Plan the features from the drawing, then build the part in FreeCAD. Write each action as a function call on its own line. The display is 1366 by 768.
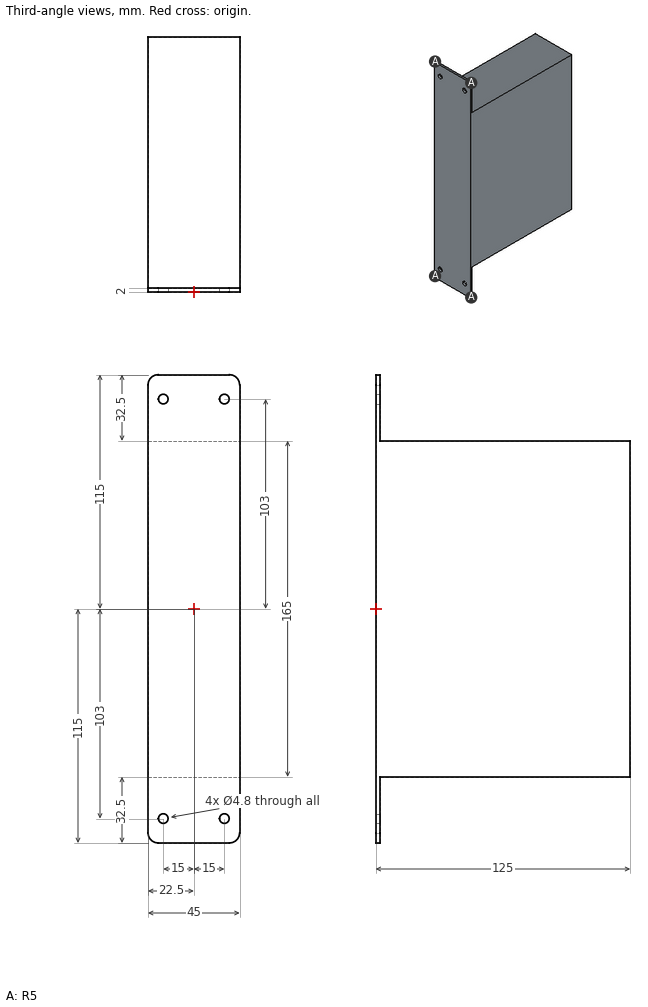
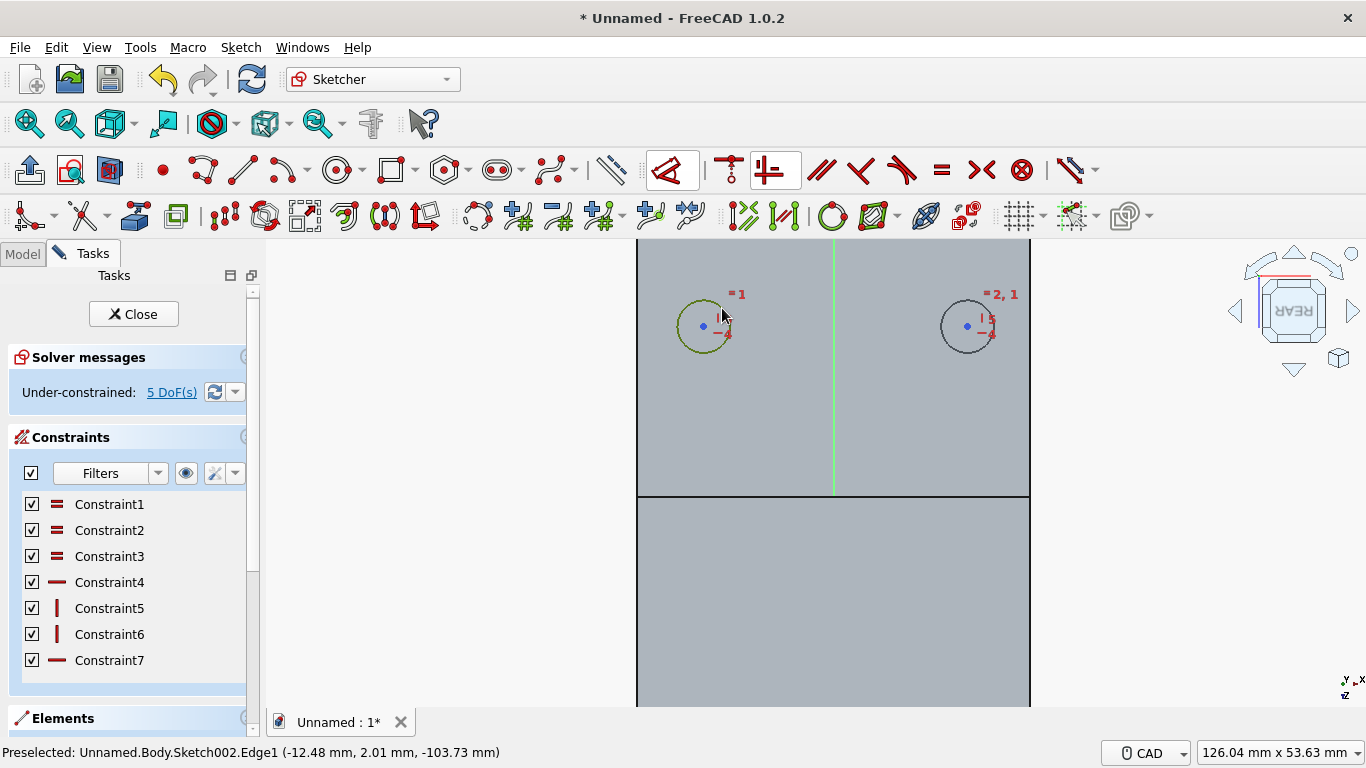
click(694, 170)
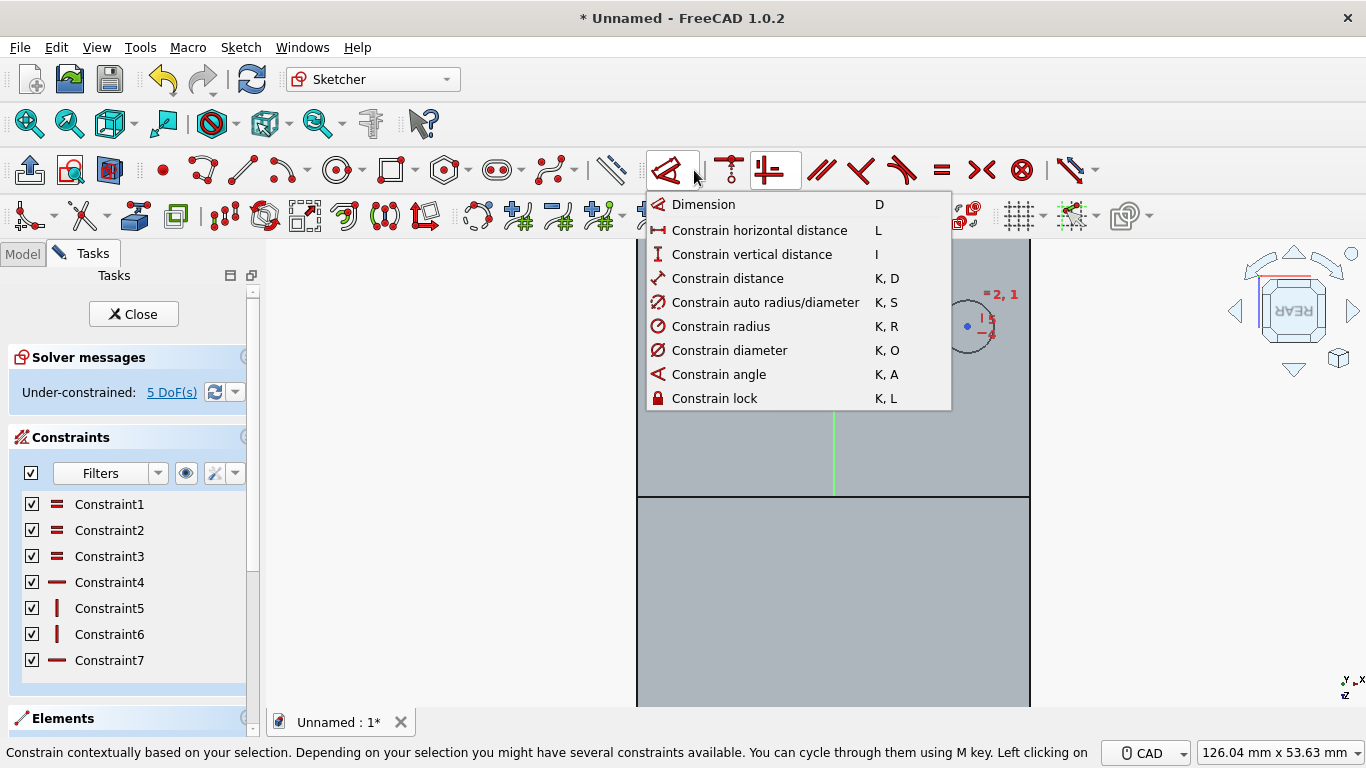
click(799, 350)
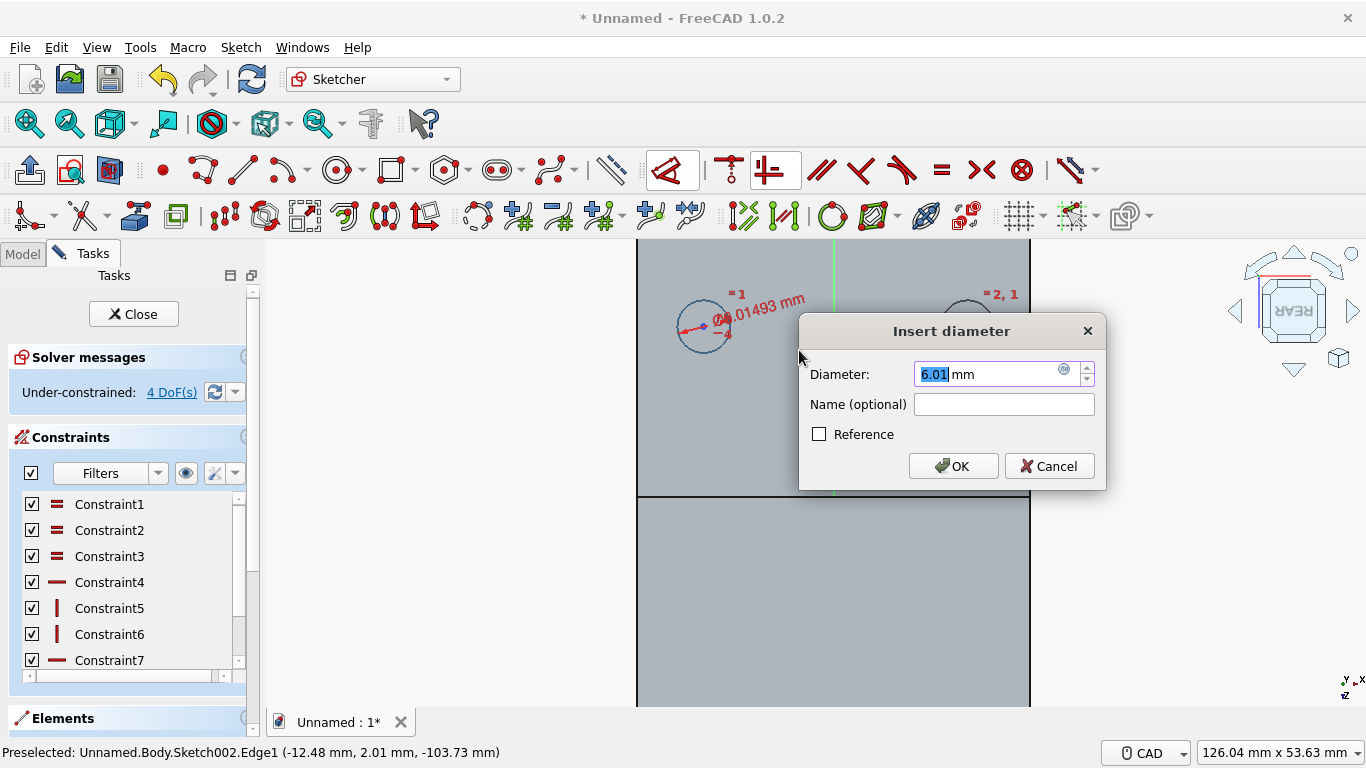
text(4.8)
key(Return)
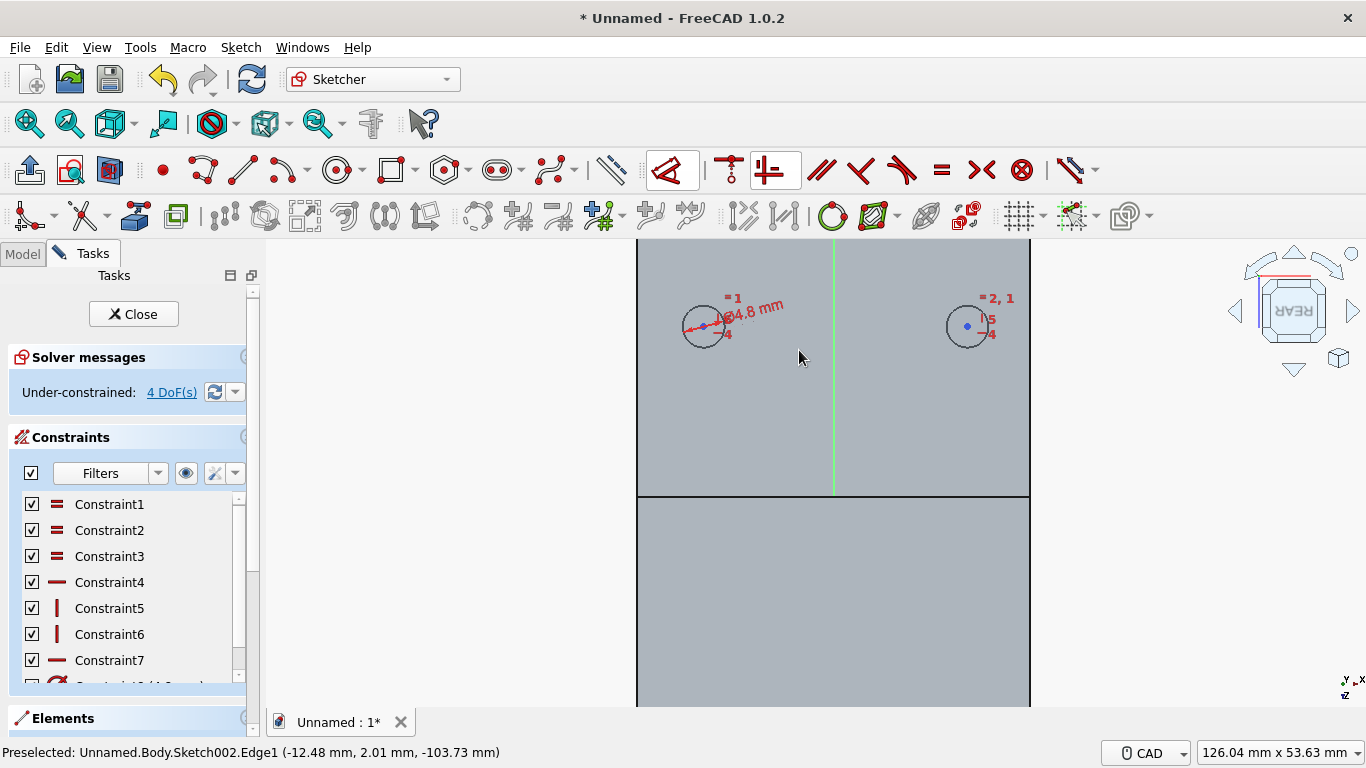
scroll(730, 326, down, 9)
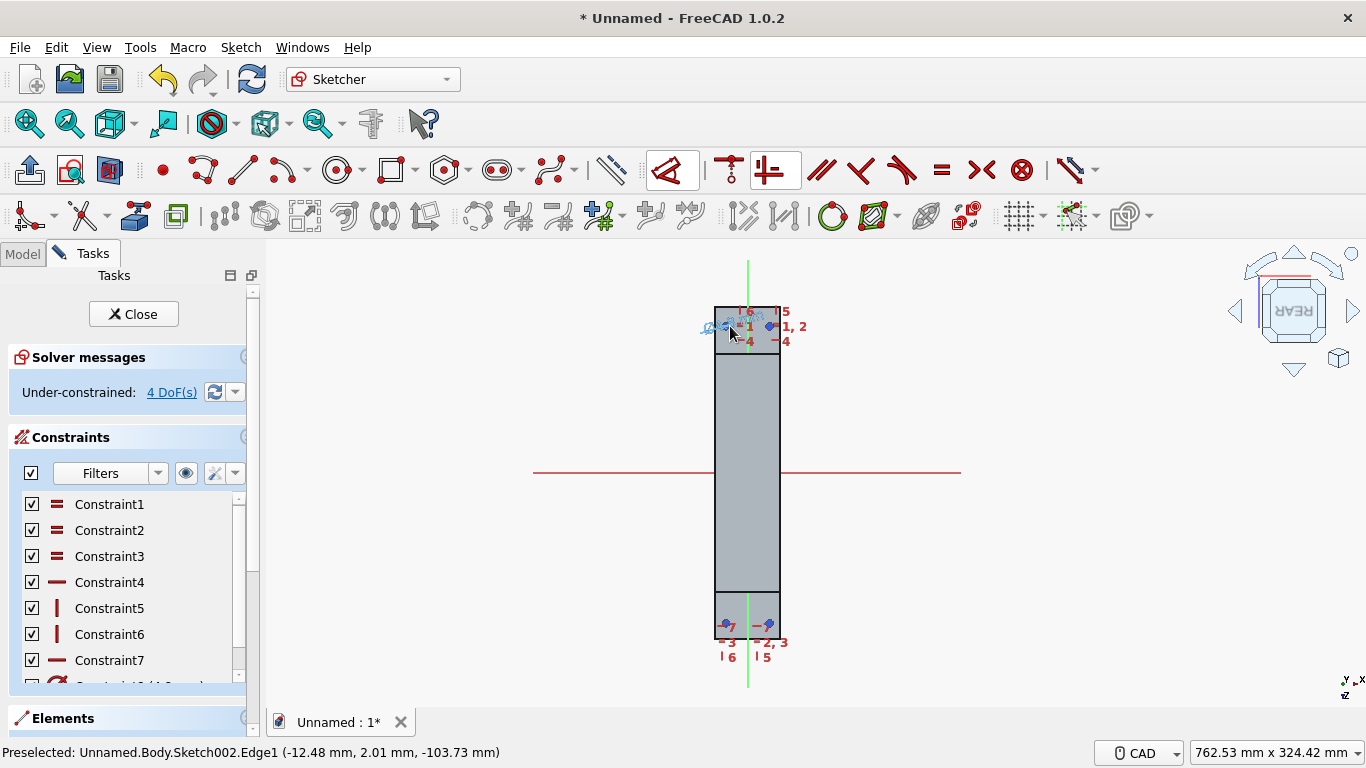
scroll(726, 326, up, 4)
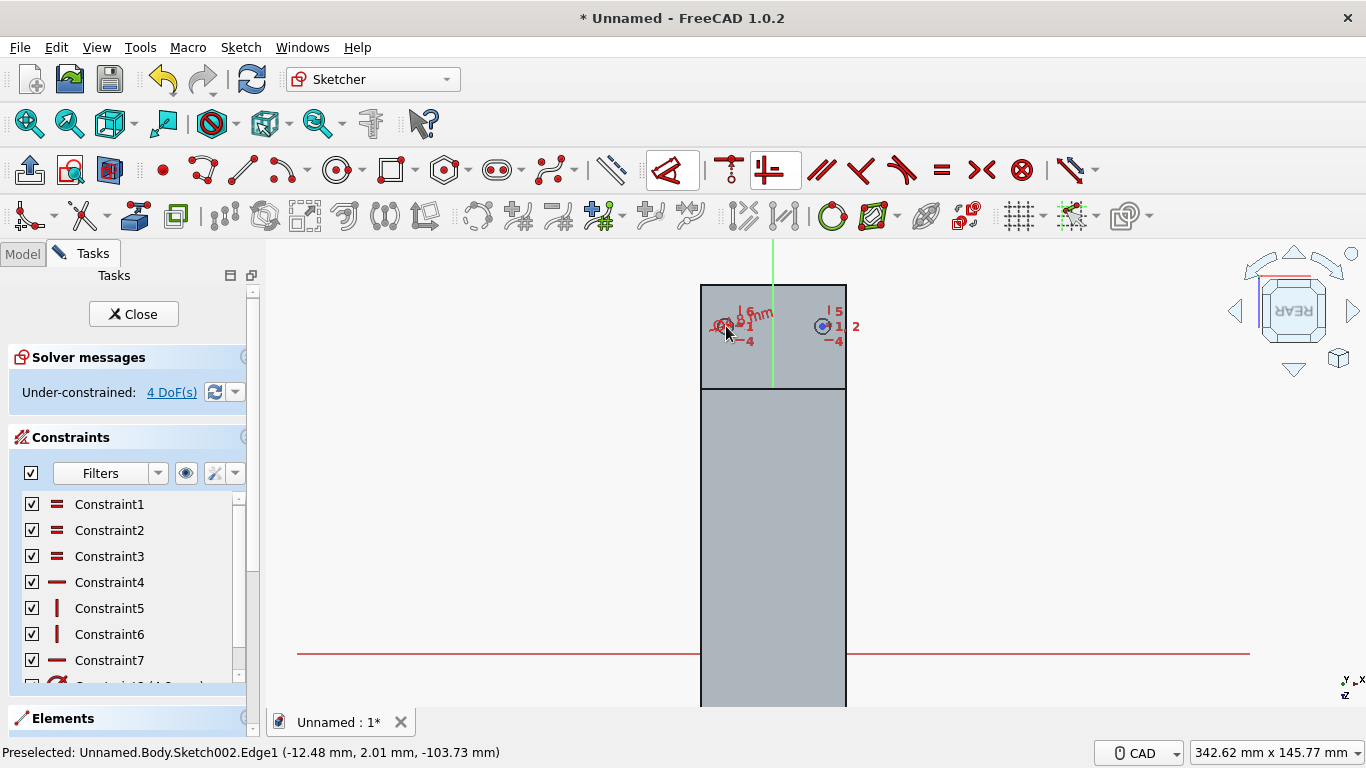
click(725, 326)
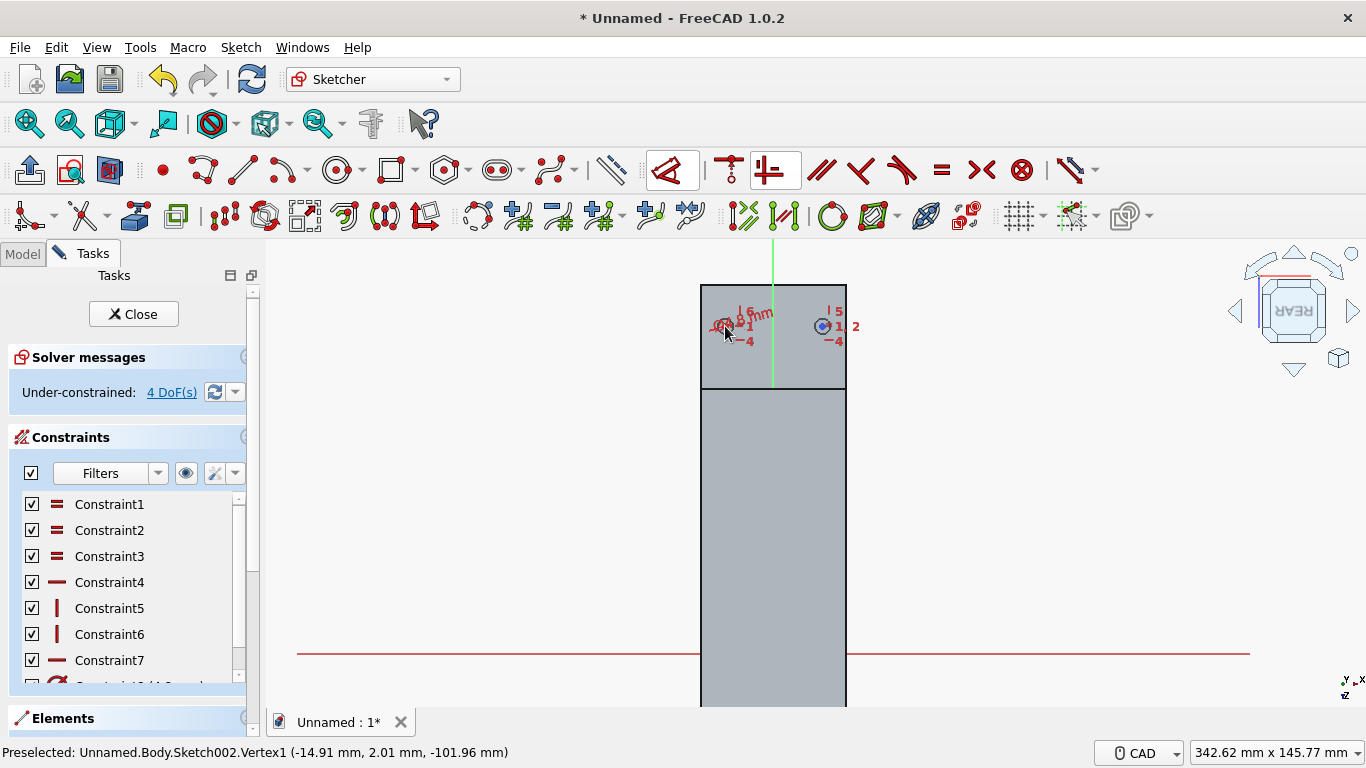
key(l)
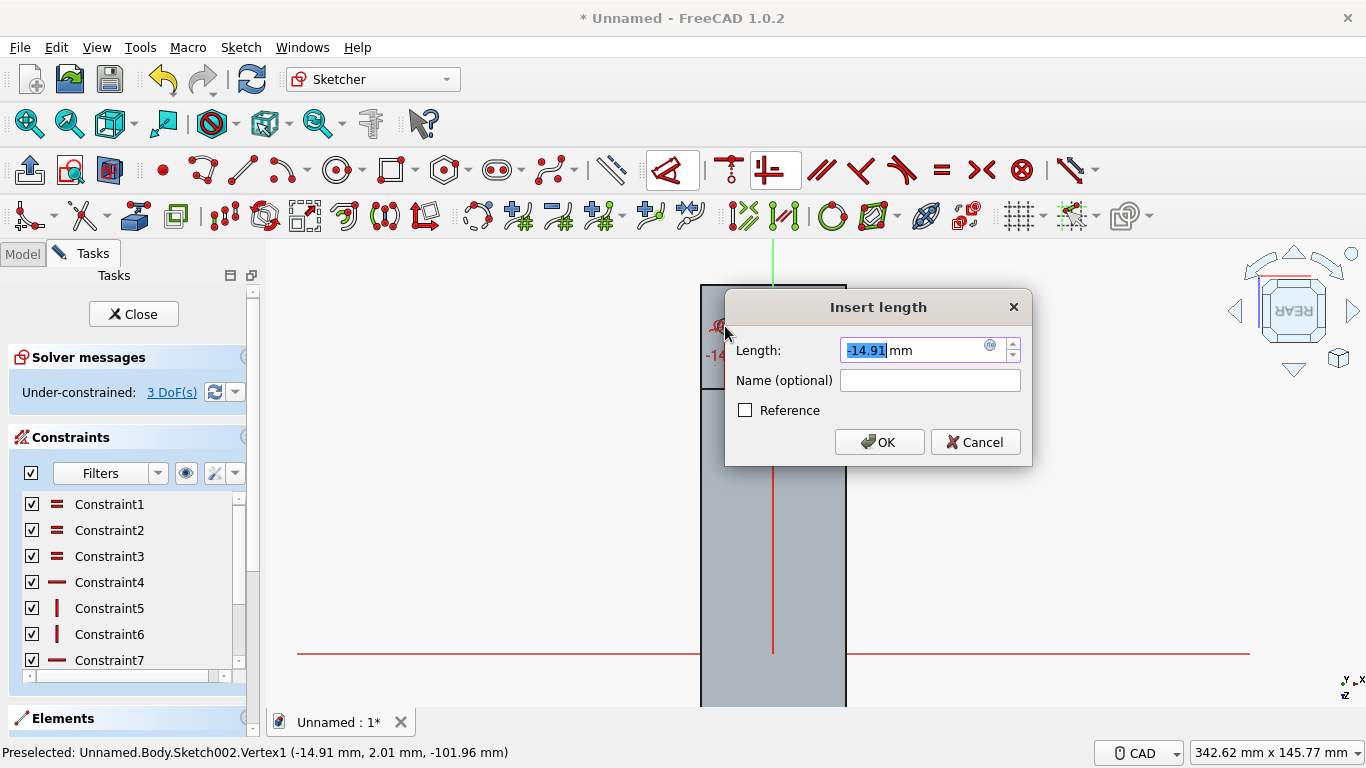
text(-15)
key(Return)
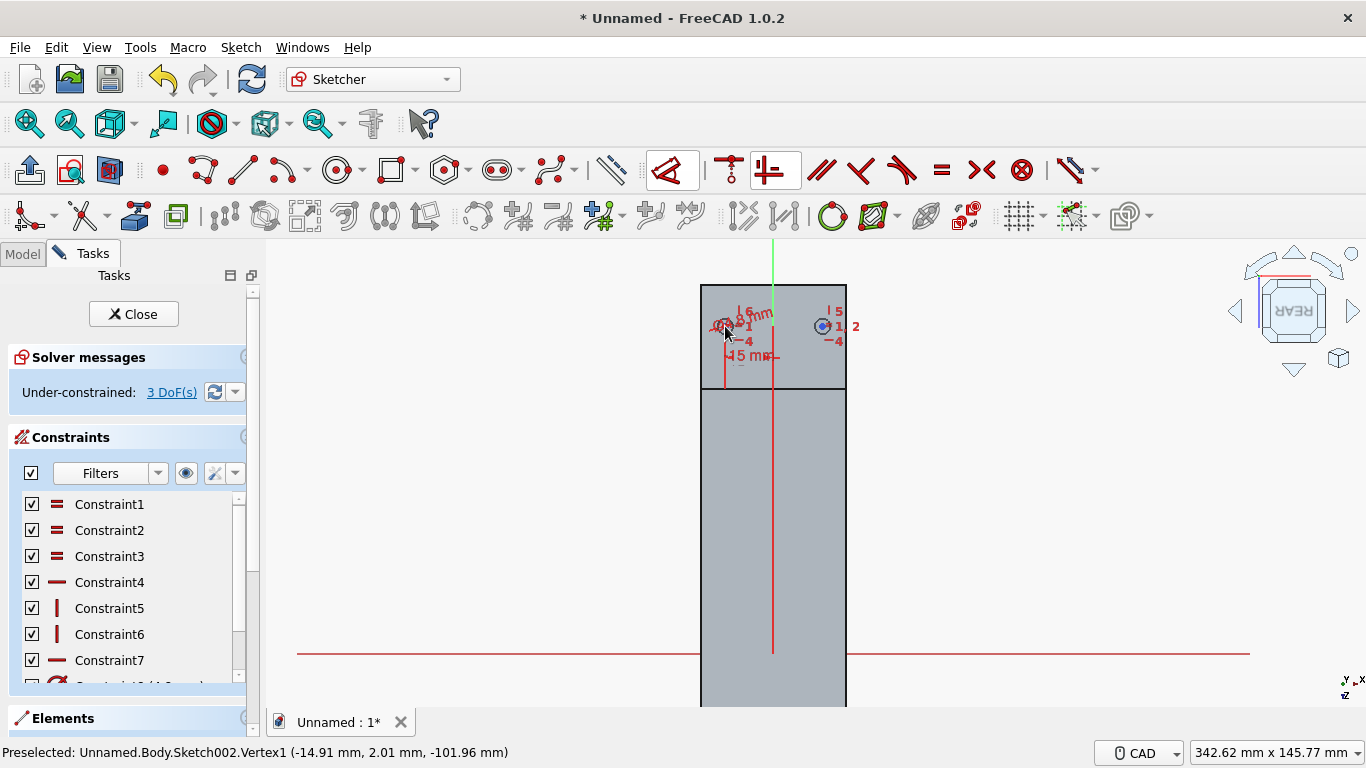
click(823, 326)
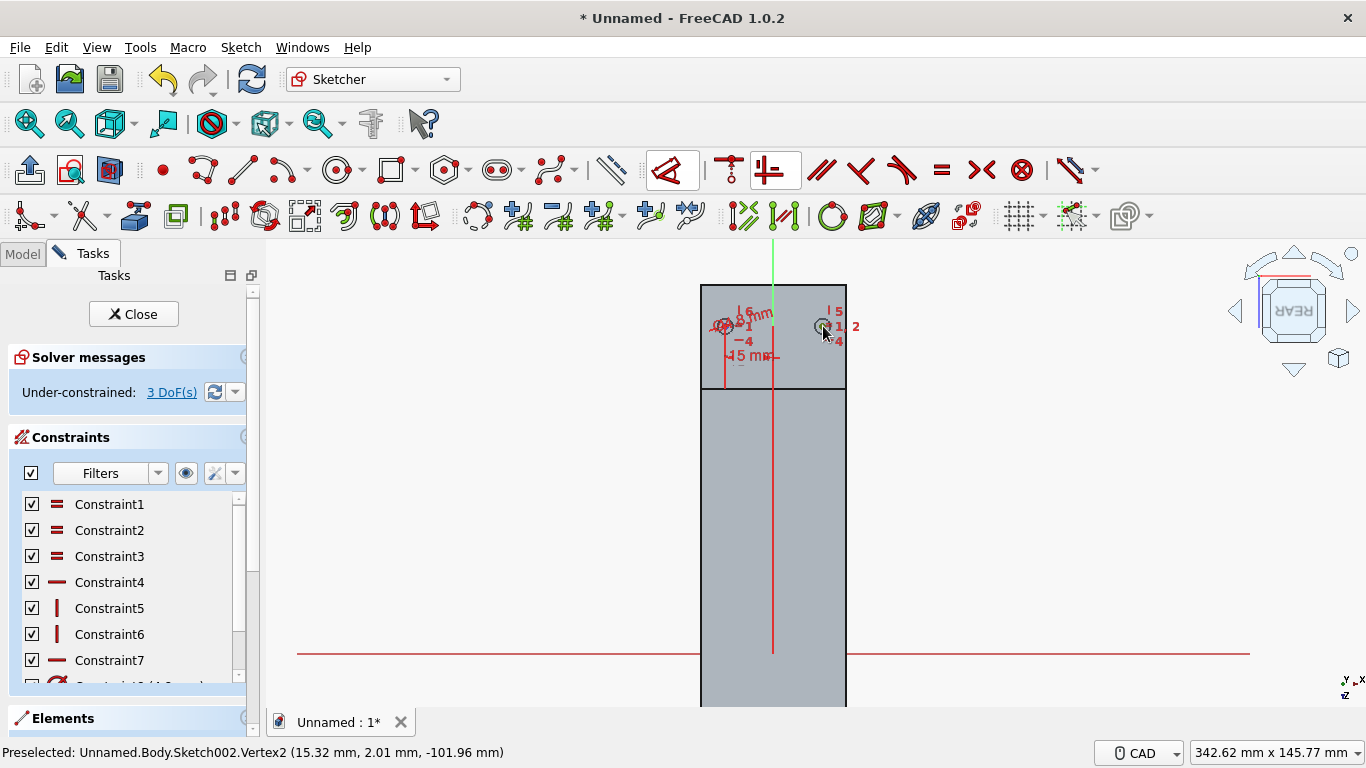
key(l)